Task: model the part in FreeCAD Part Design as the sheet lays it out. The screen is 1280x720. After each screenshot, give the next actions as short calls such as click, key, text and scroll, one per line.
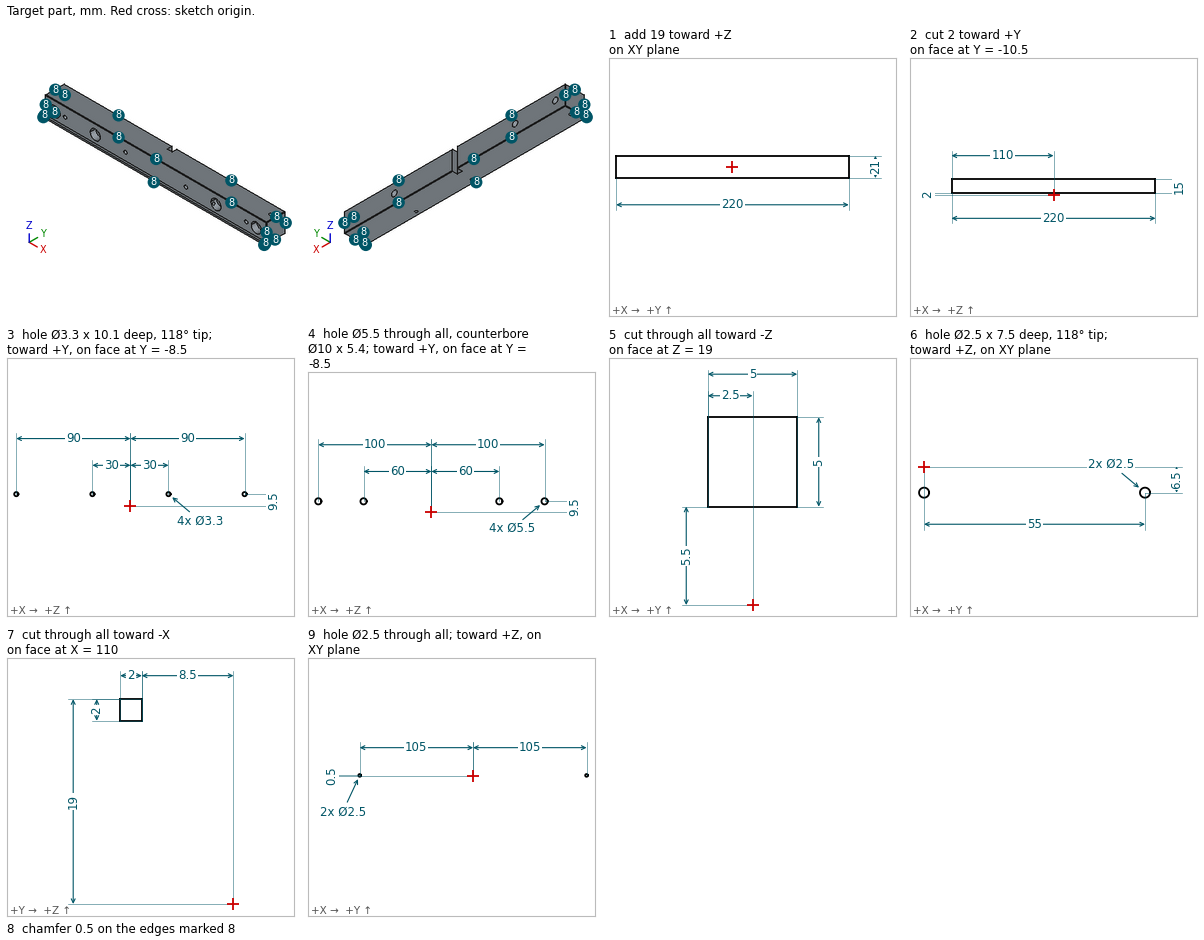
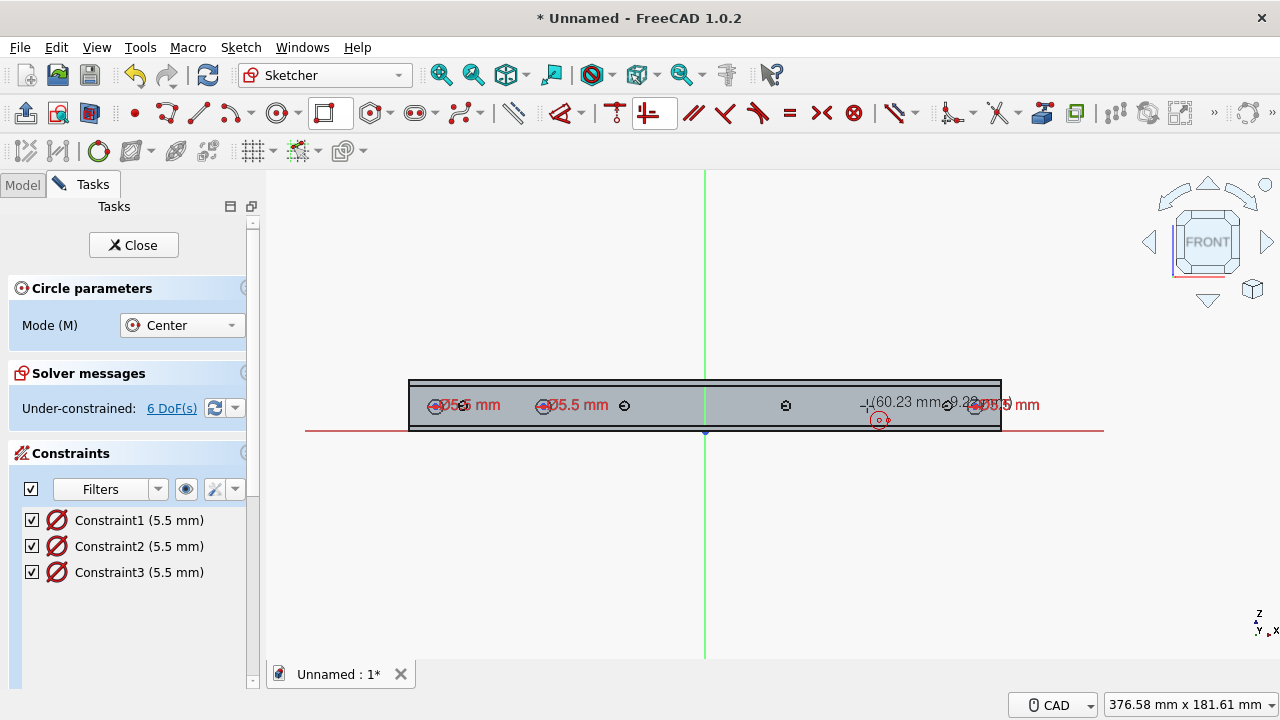
click(867, 406)
move(872, 401)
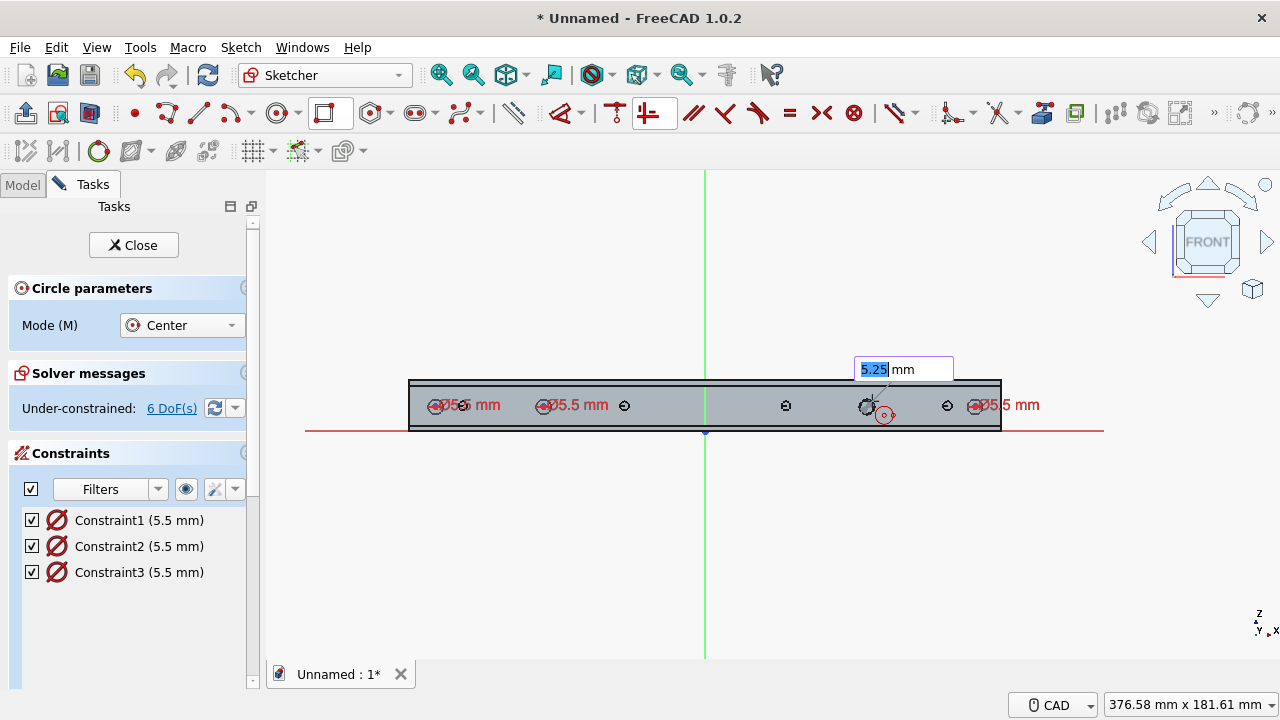
text(5.5)
key(Return)
key(Escape)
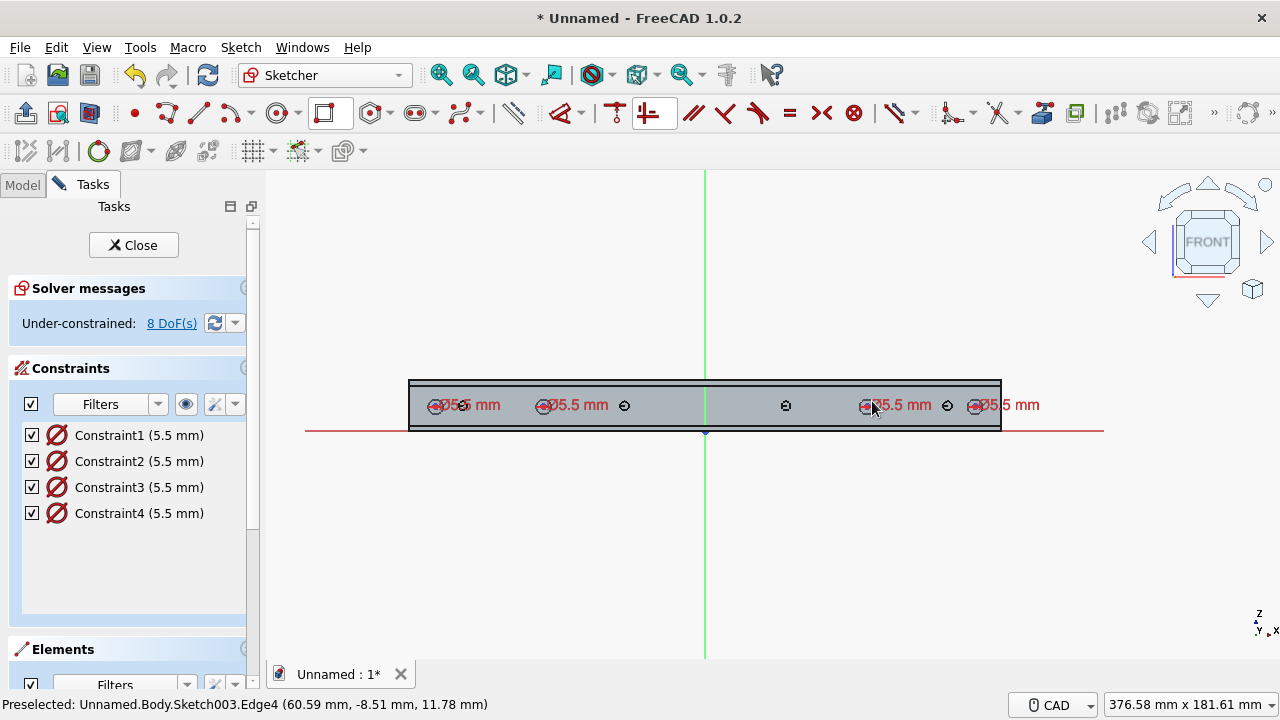
click(975, 407)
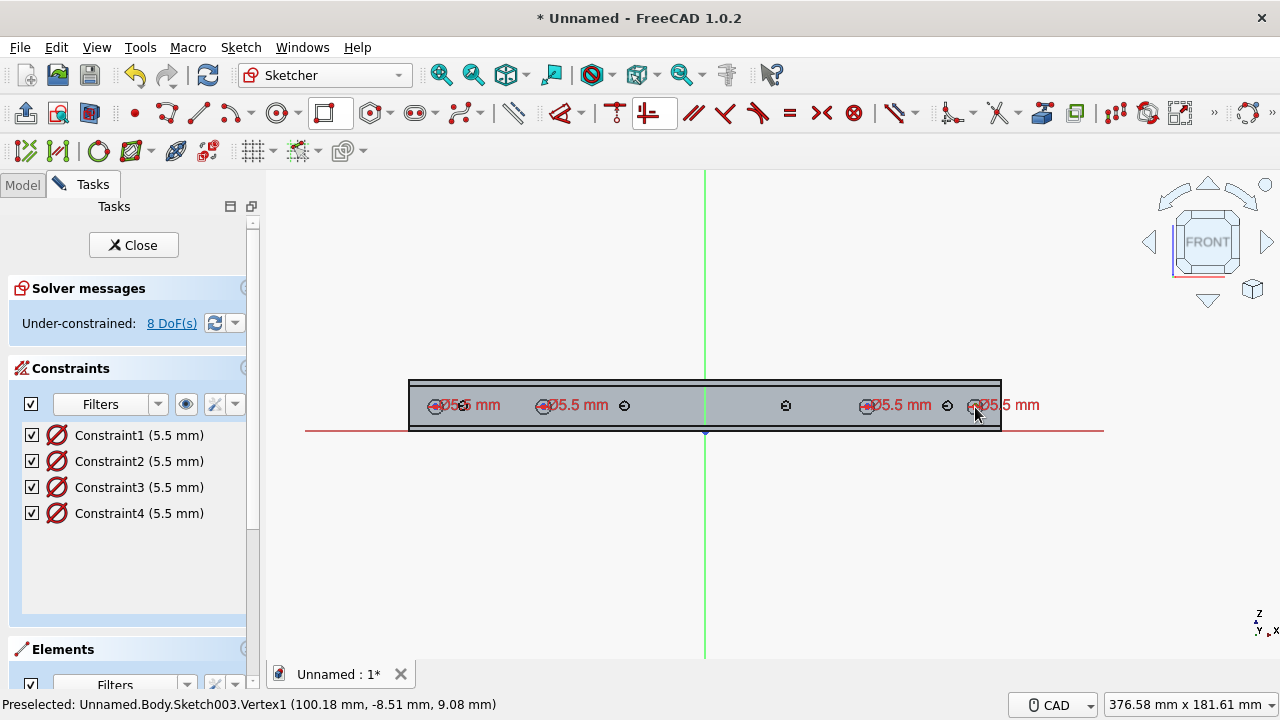
click(436, 407)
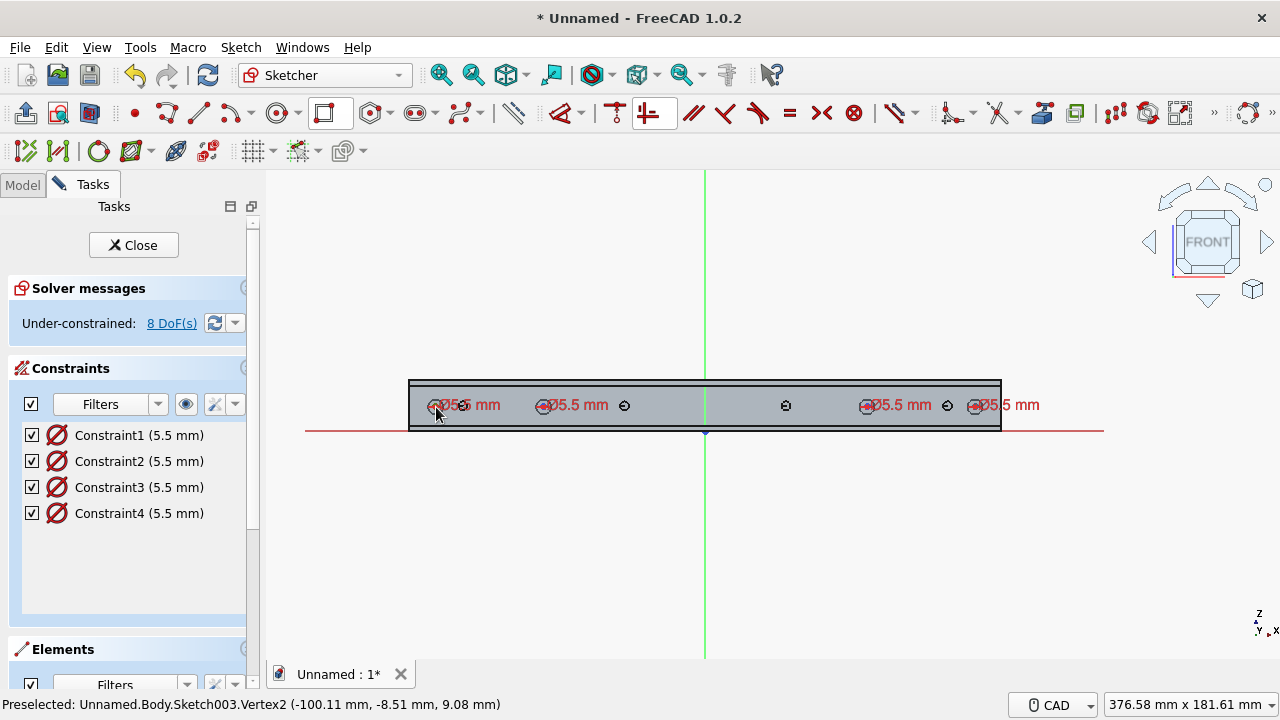
key(h)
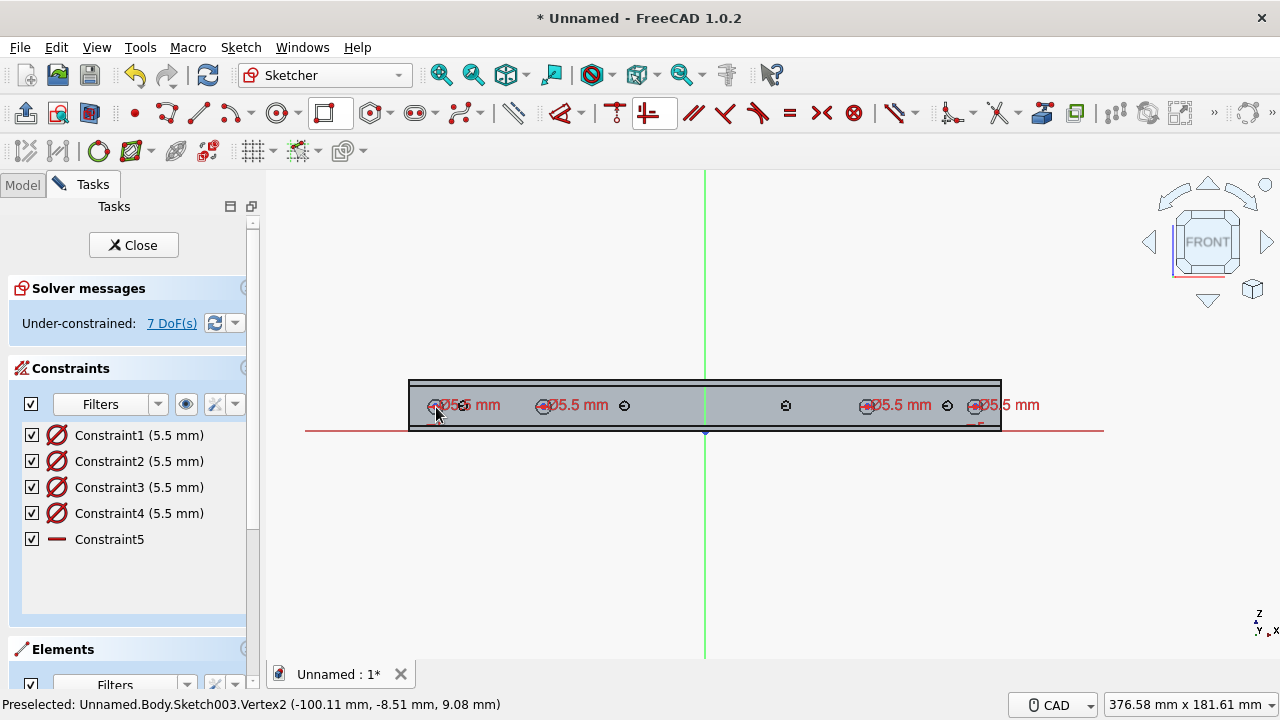
click(436, 407)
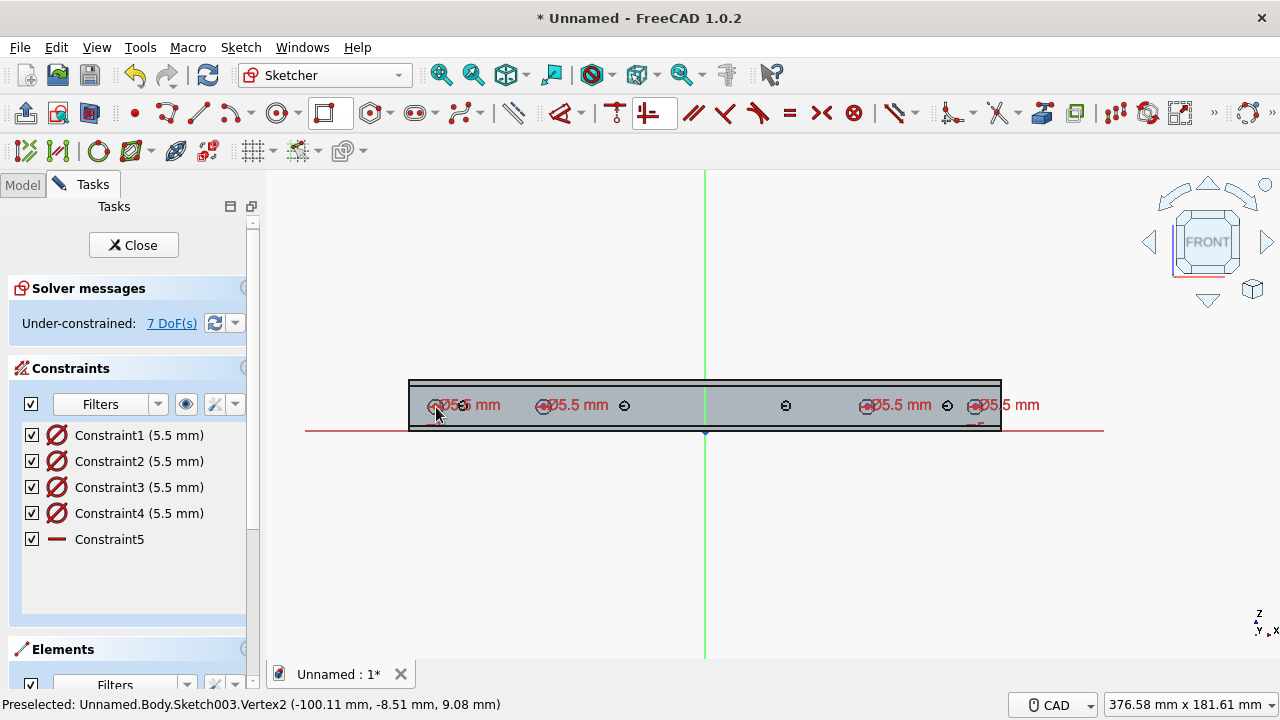
click(544, 407)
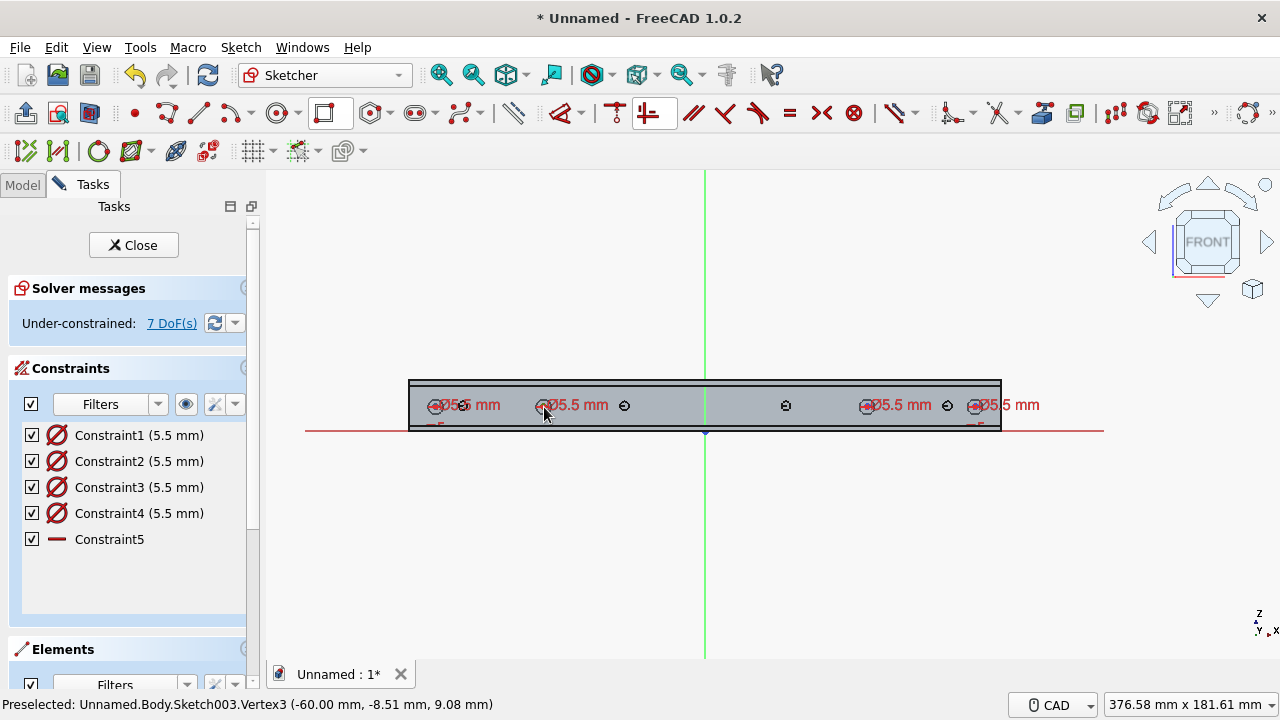
key(h)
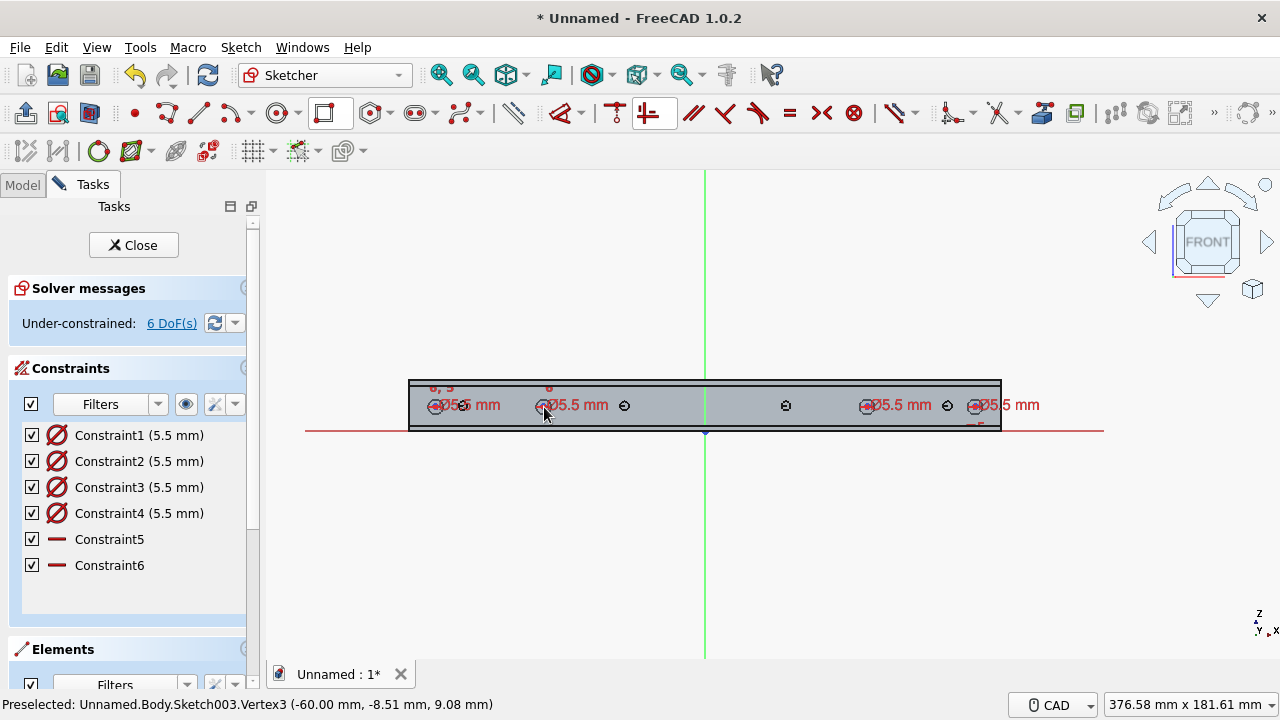
click(975, 407)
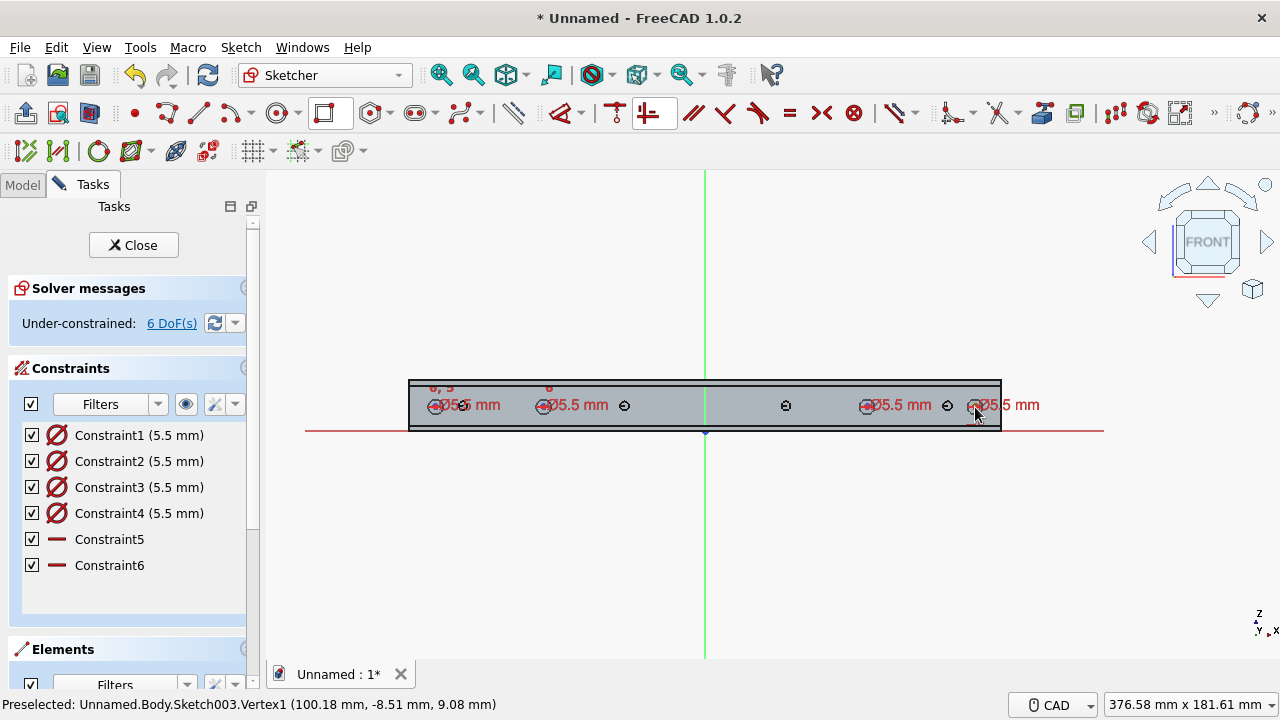
click(867, 407)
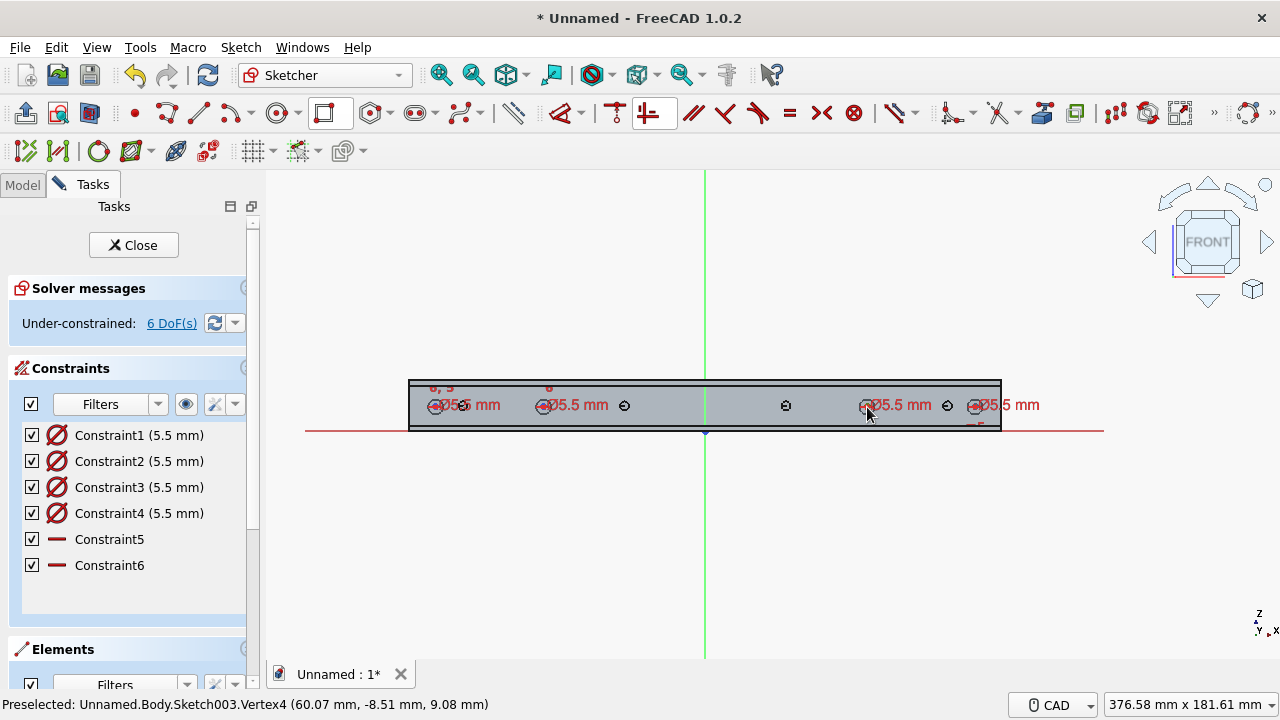
key(h)